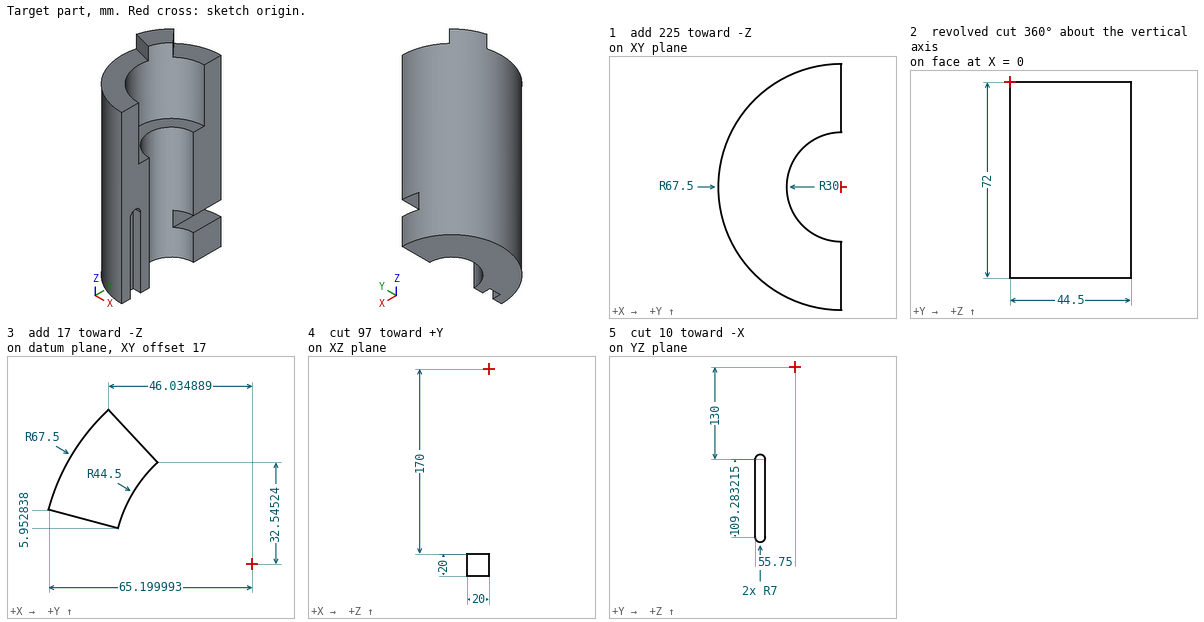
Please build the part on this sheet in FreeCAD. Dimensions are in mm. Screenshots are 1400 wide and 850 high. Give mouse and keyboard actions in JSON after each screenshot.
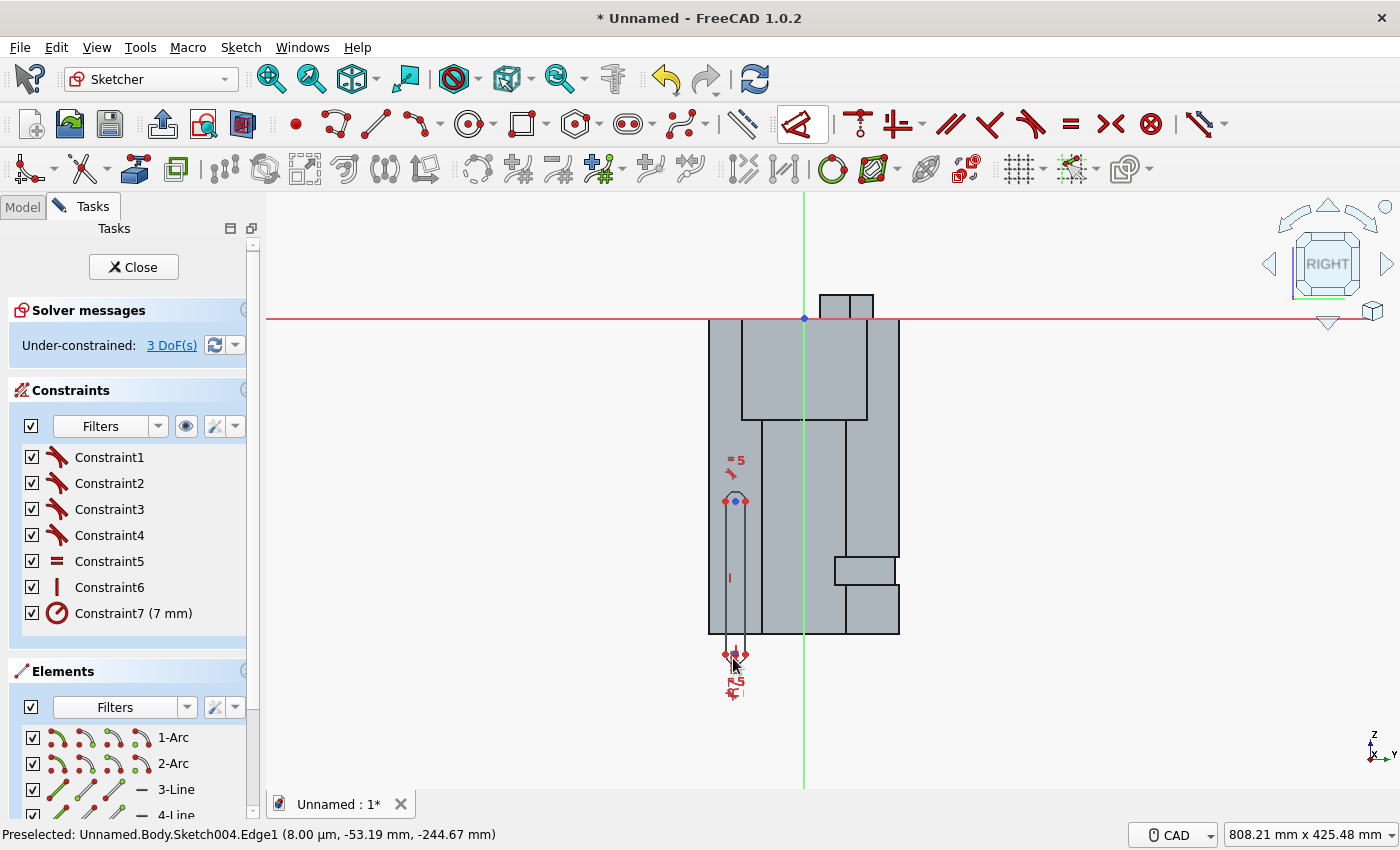
{"action": "scroll", "coordinate": [745, 501], "scroll_direction": "up", "scroll_amount": 2}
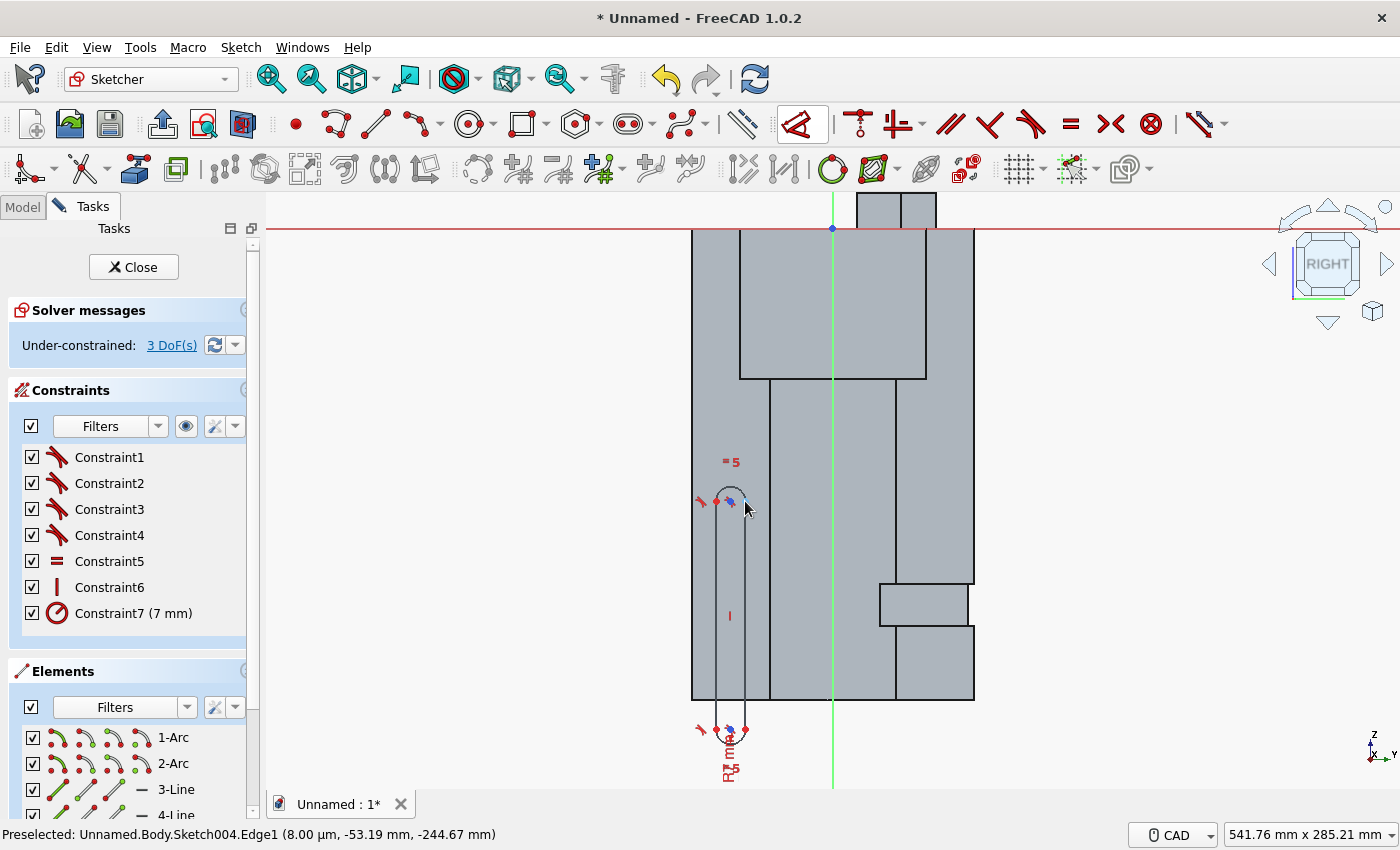
{"action": "left_click", "coordinate": [745, 501]}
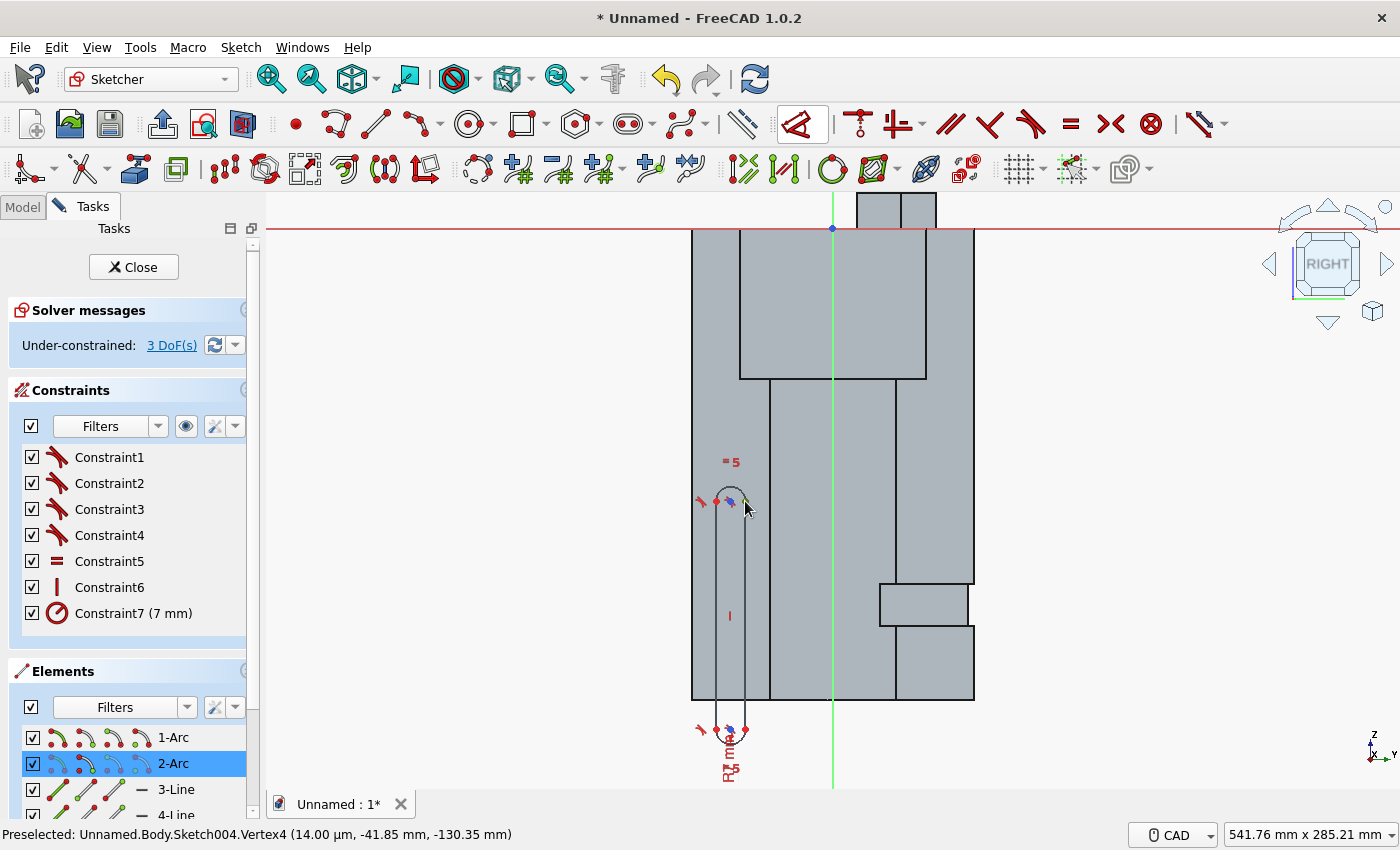
{"action": "key", "text": "i"}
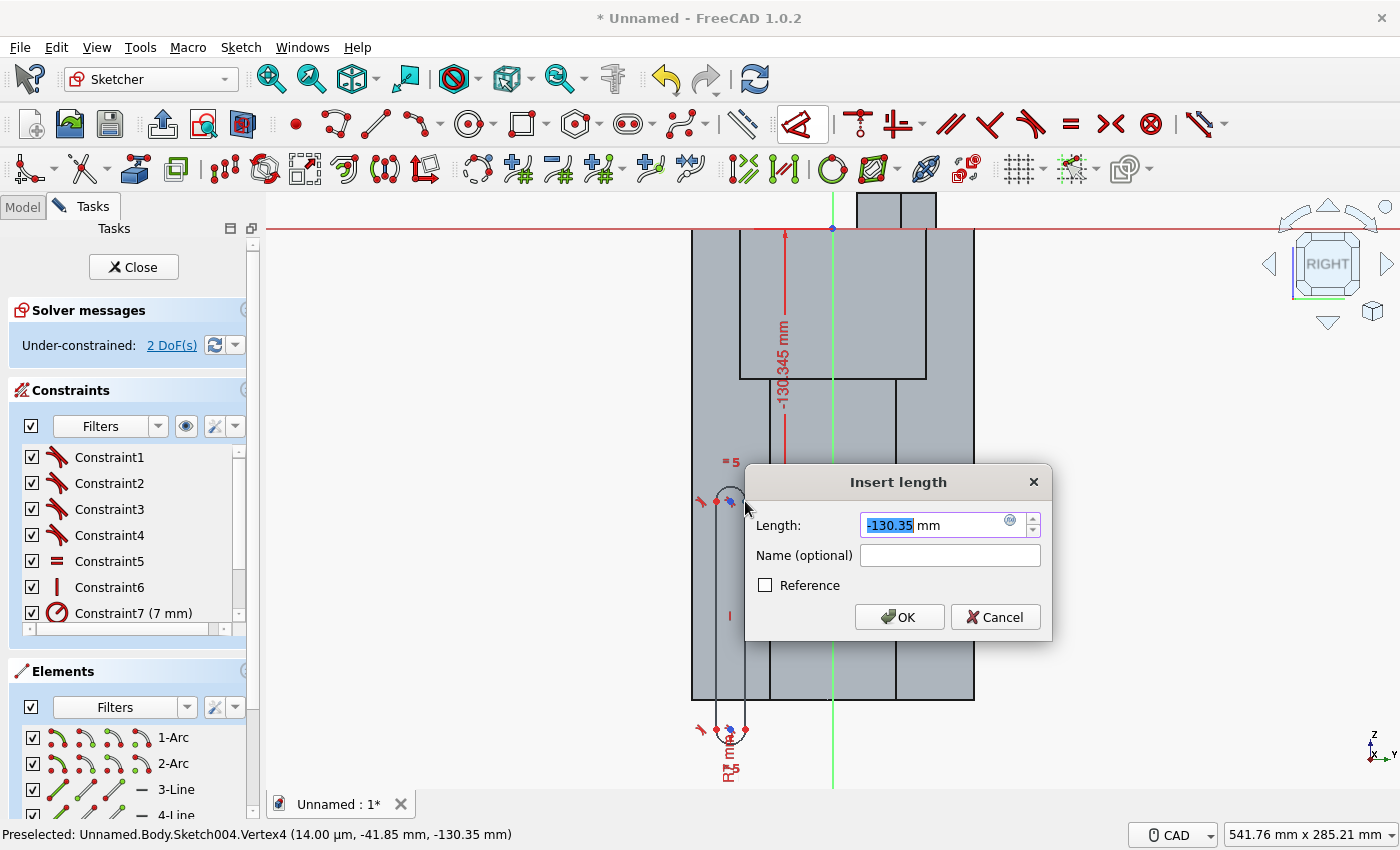
{"action": "type", "text": "-130"}
{"action": "key", "text": "Return"}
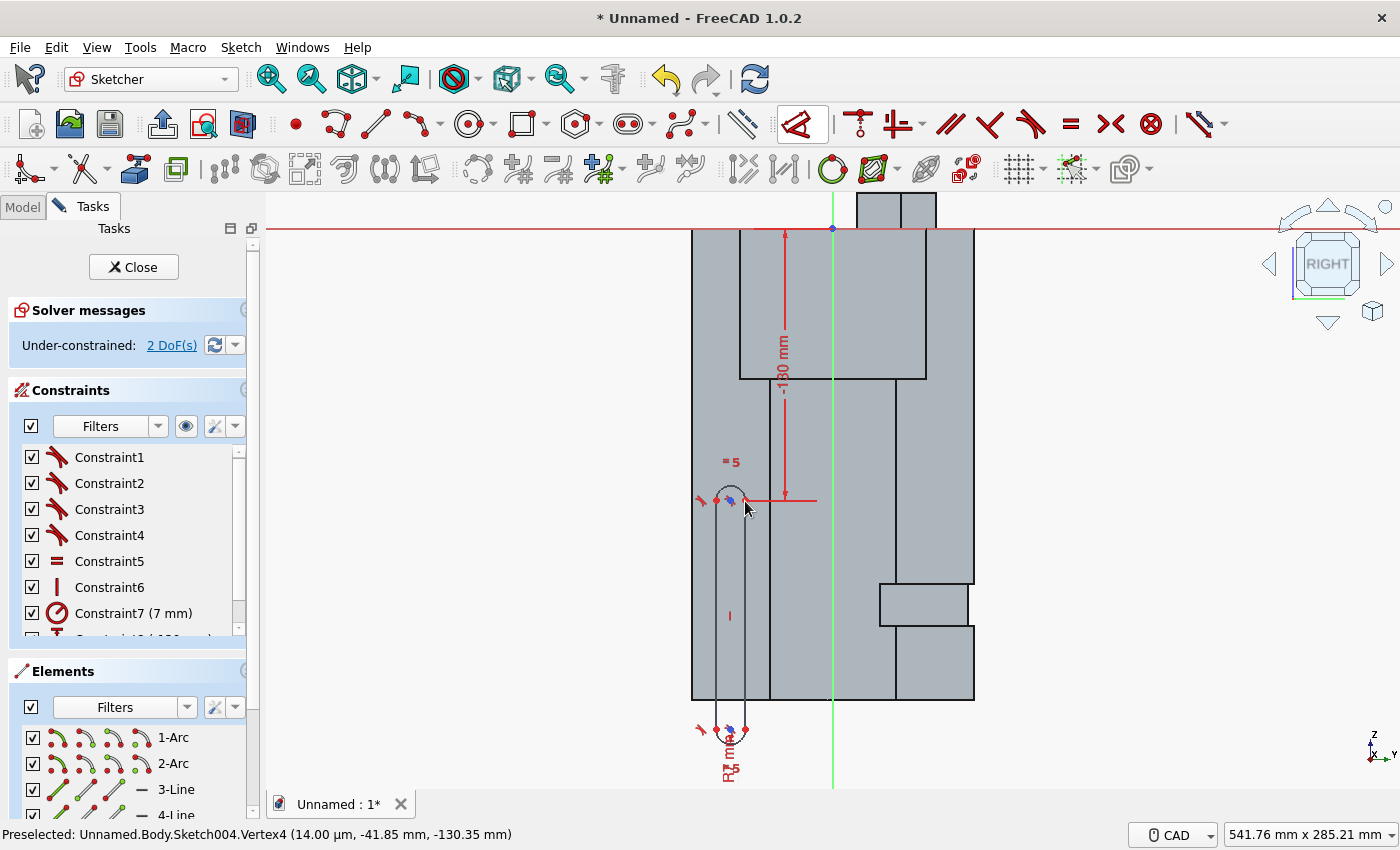
{"action": "left_click", "coordinate": [716, 730]}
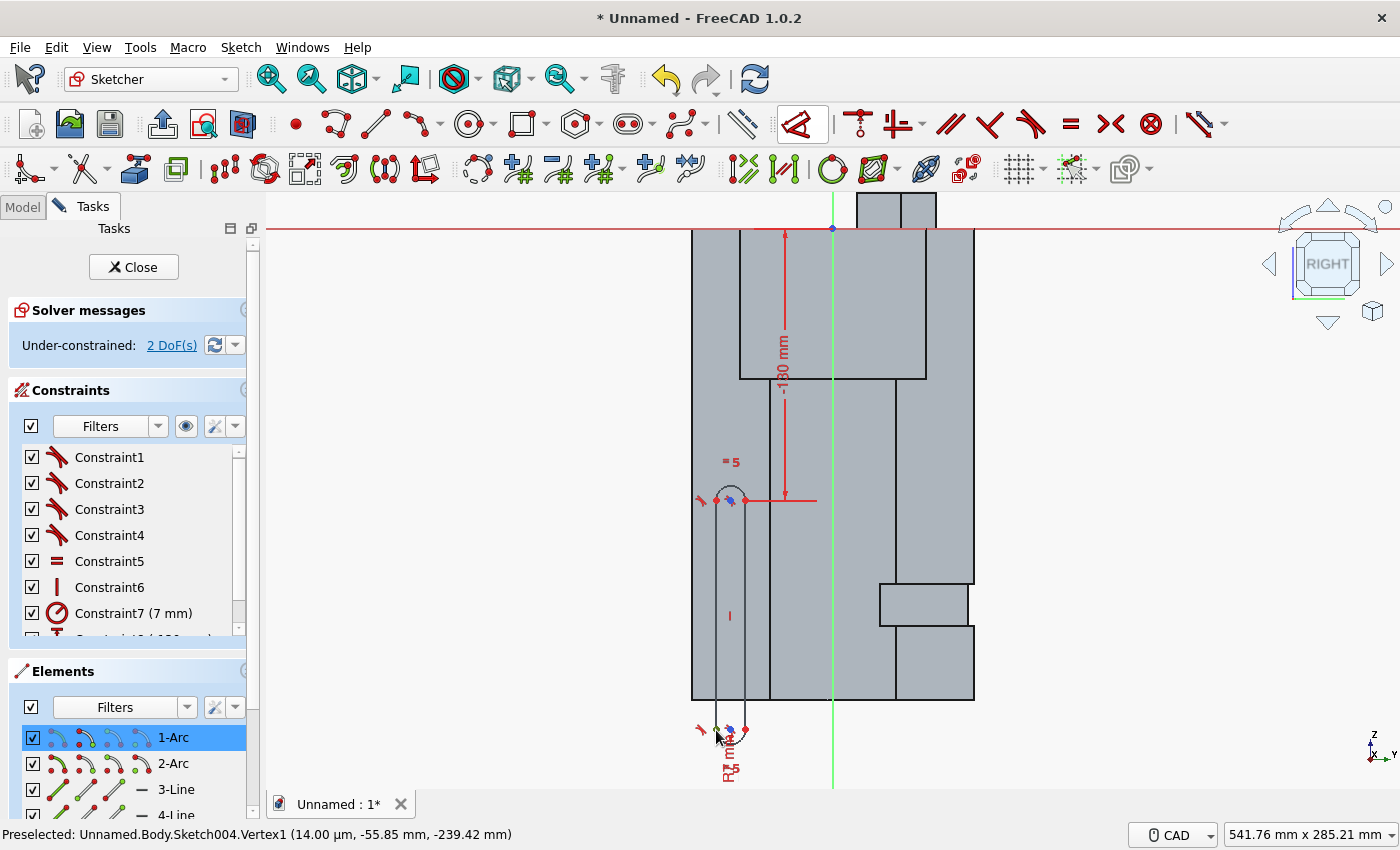
{"action": "key", "text": "l"}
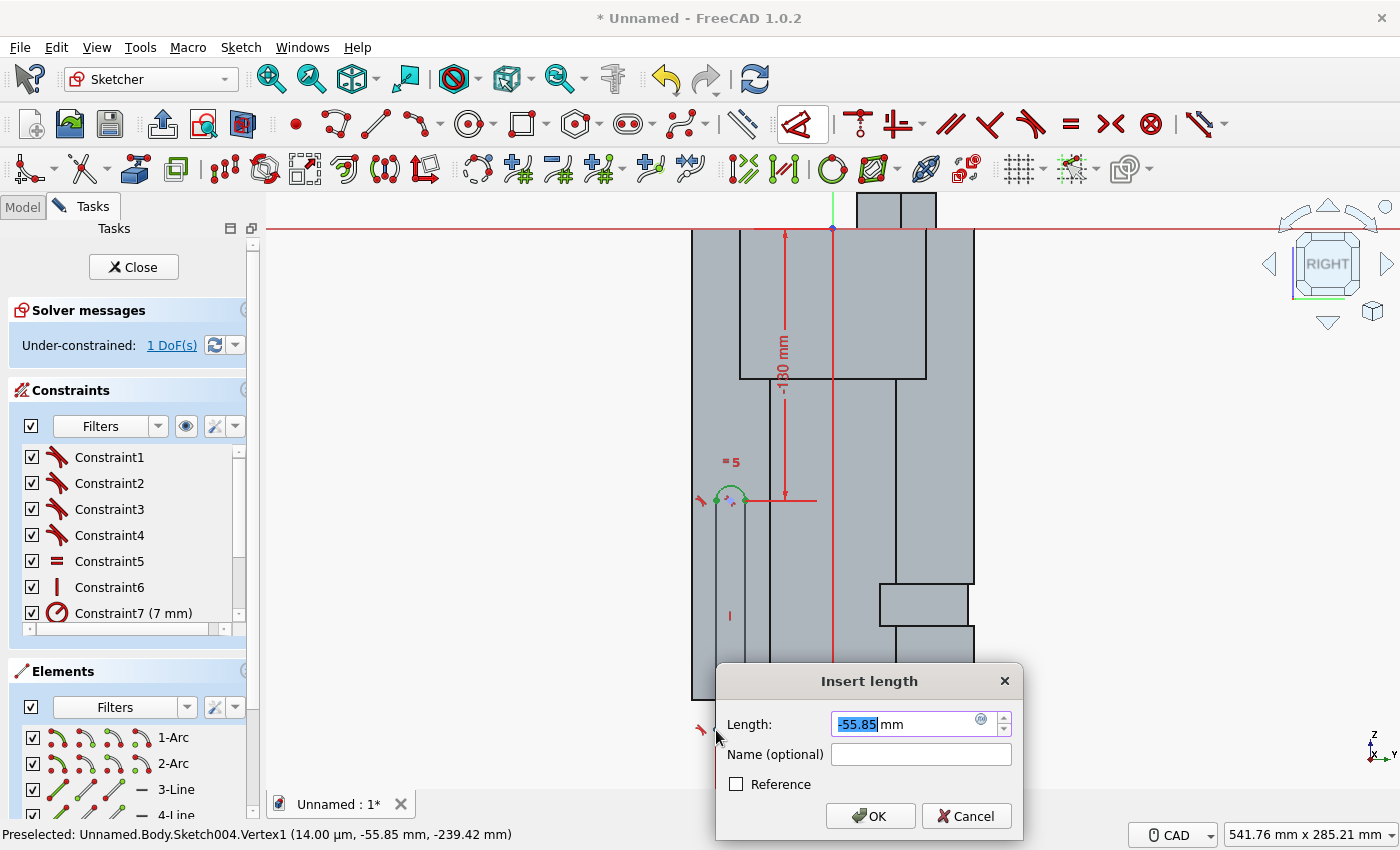
{"action": "type", "text": "-55.75"}
{"action": "key", "text": "Return"}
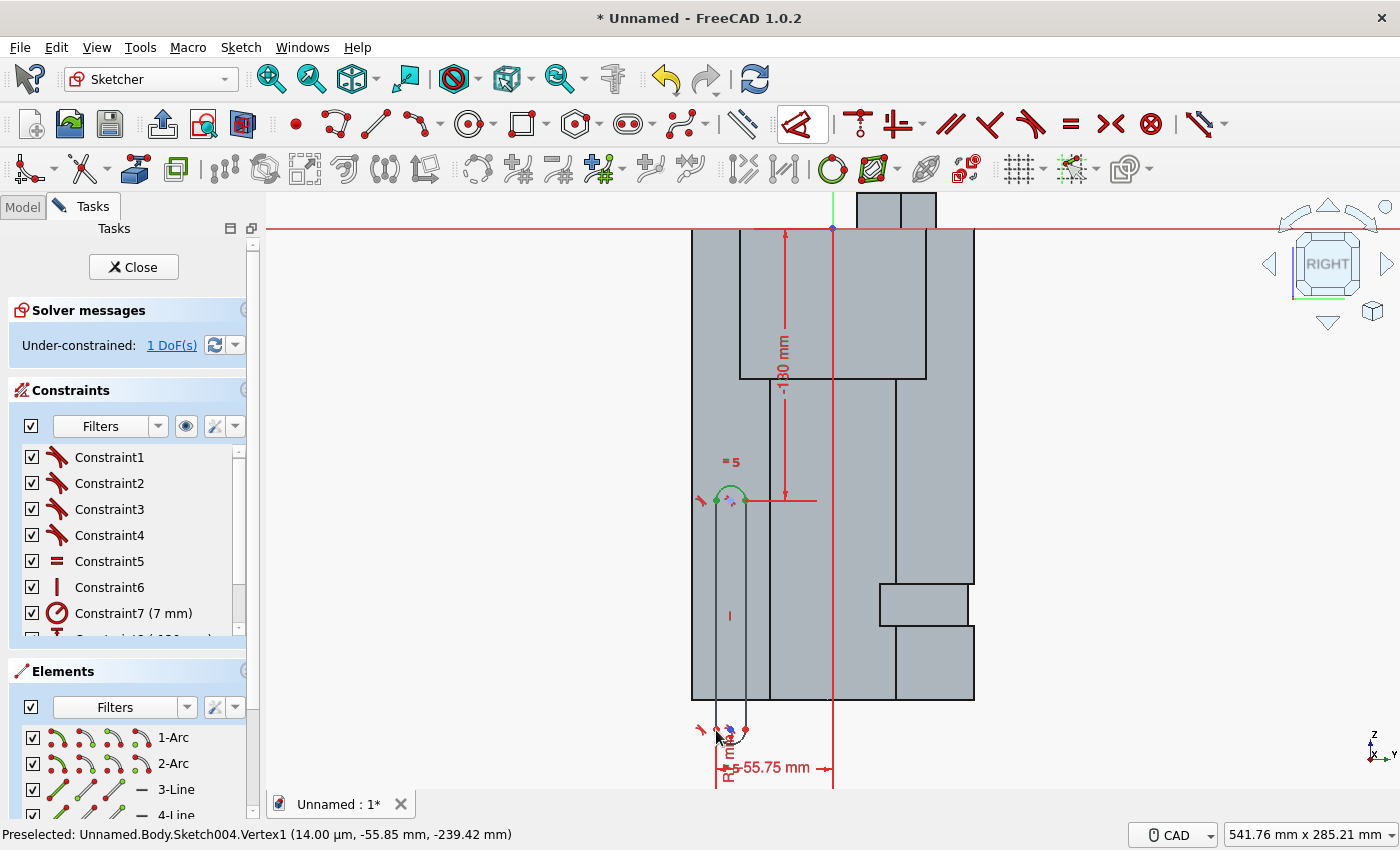
{"action": "left_click", "coordinate": [716, 661]}